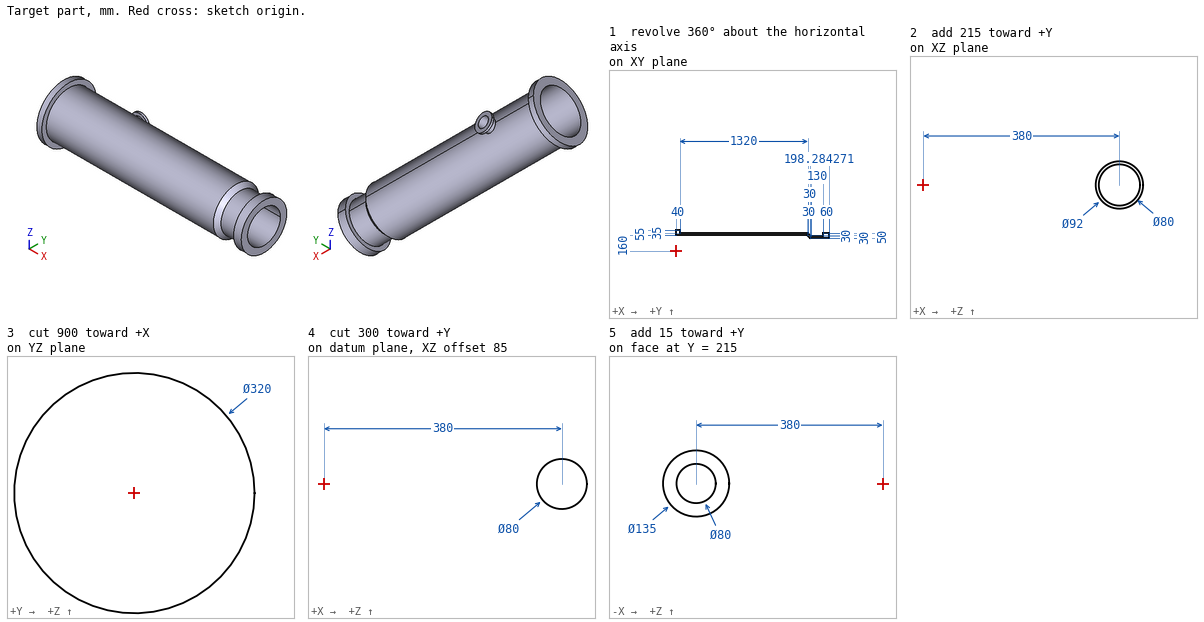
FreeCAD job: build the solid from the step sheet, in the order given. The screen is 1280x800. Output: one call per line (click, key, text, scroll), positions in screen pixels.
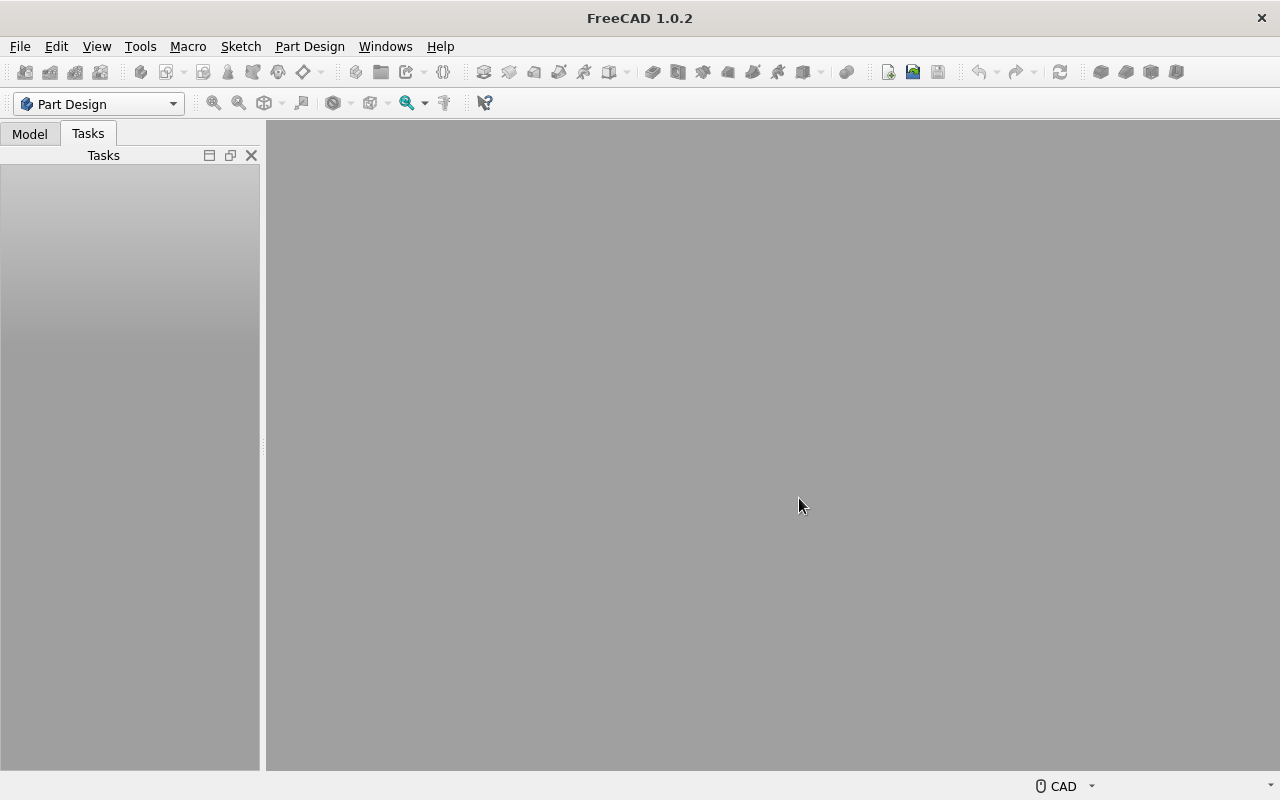
key(ctrl+n)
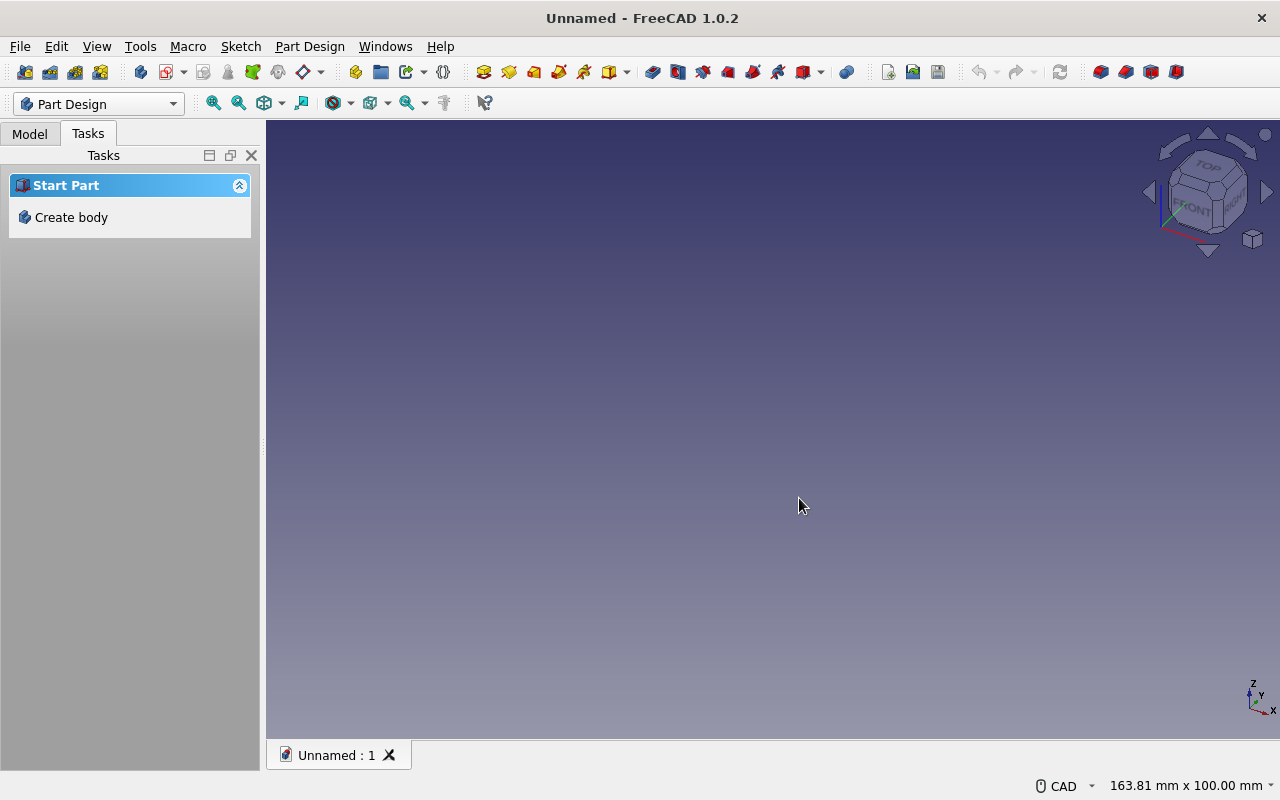
click(166, 72)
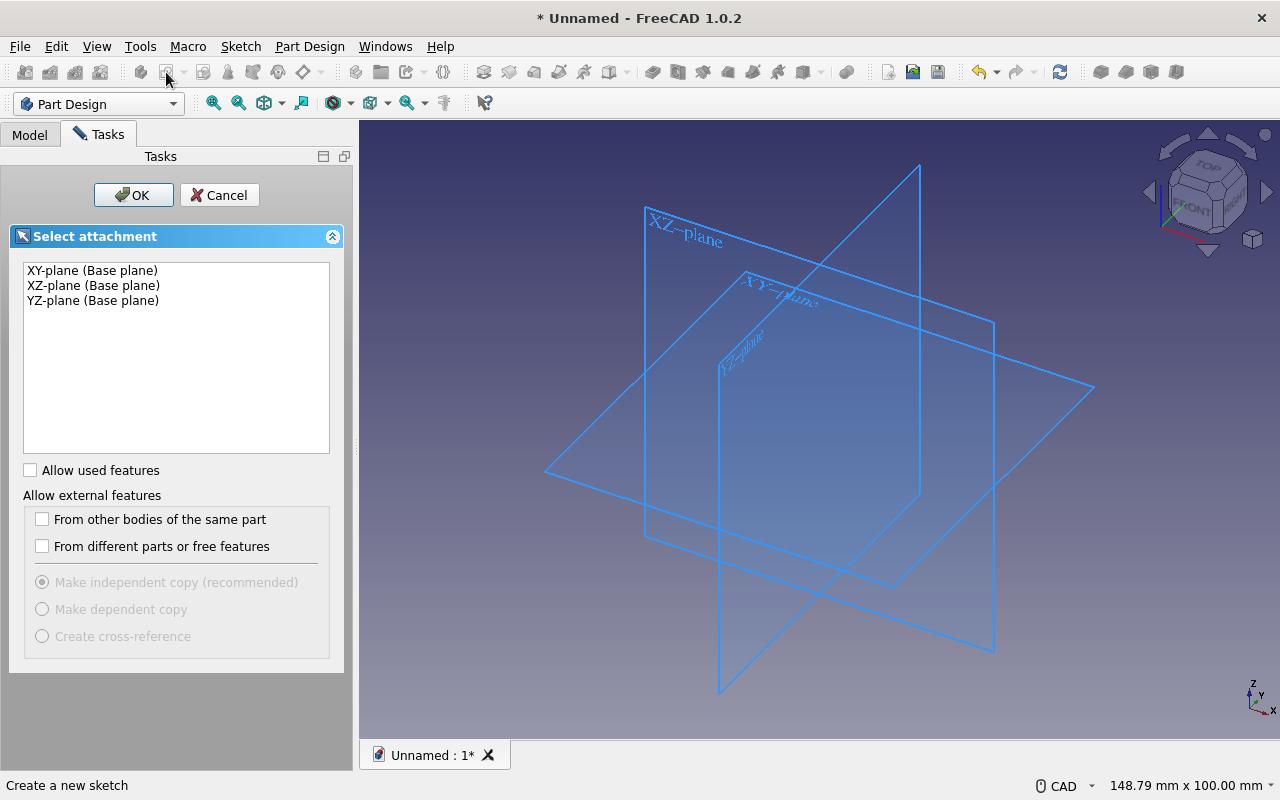
click(84, 270)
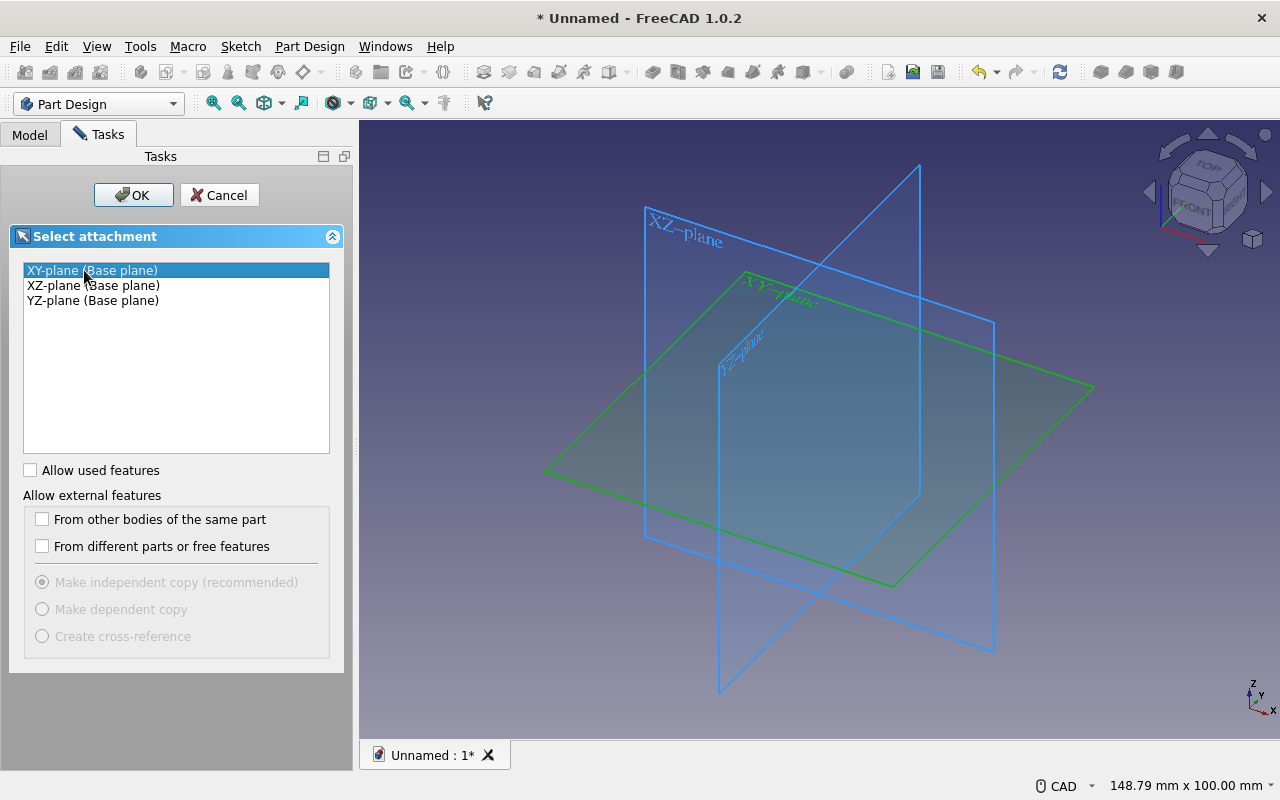
click(134, 195)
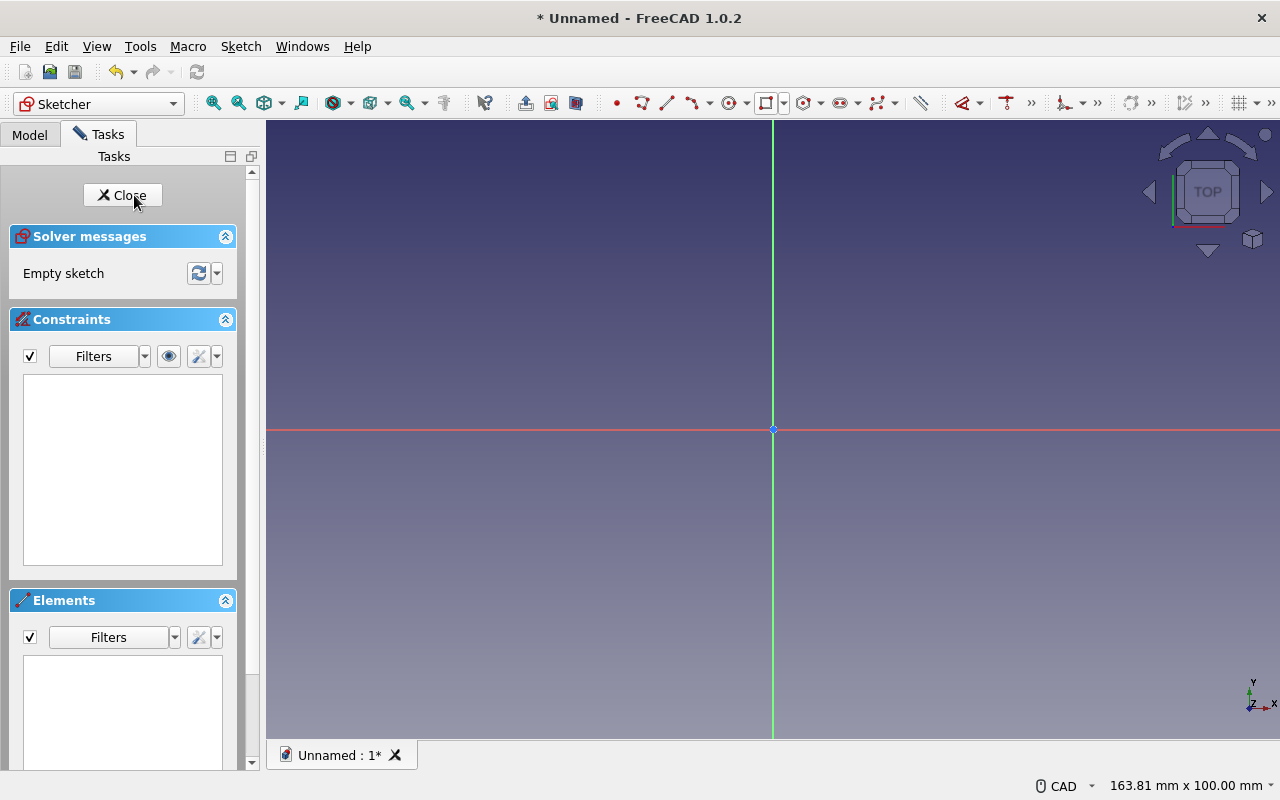
scroll(383, 473, down, 14)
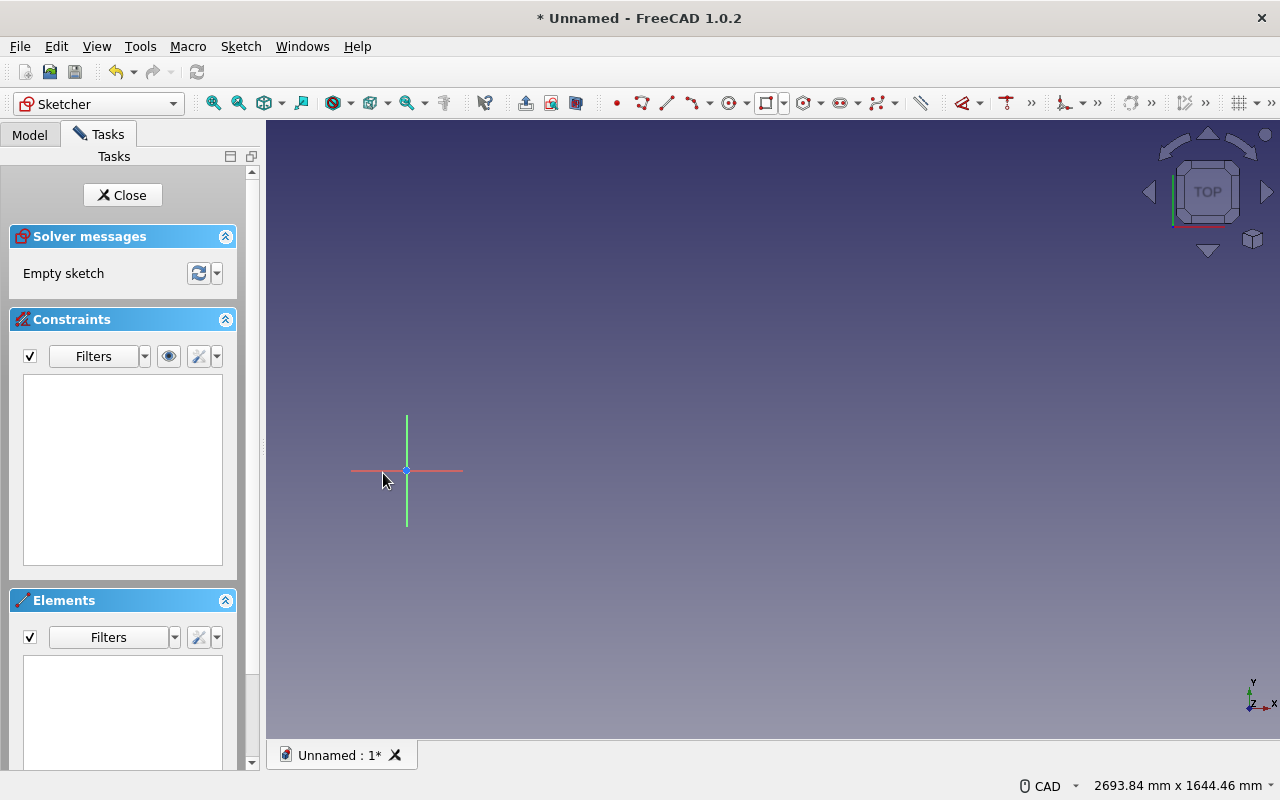
key(g)
key(m)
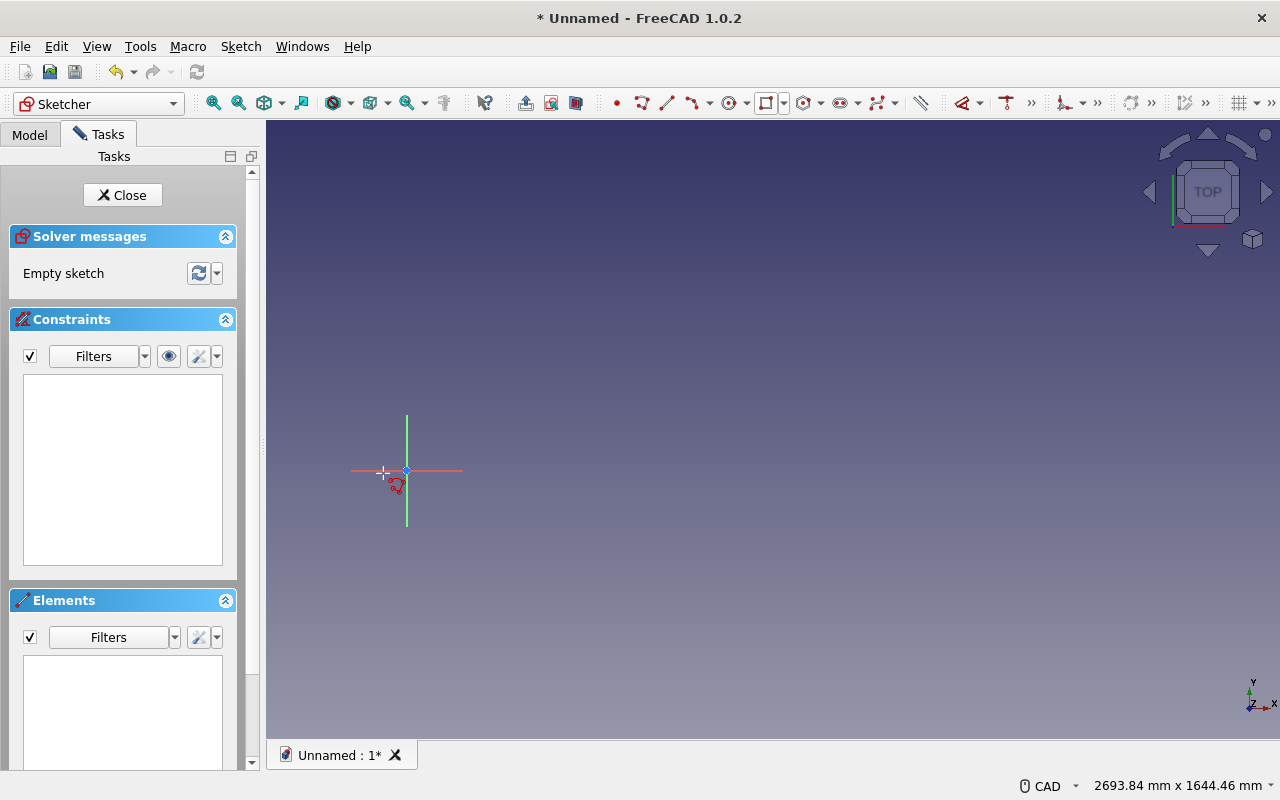
click(407, 411)
click(916, 411)
click(927, 422)
click(1002, 422)
click(1002, 403)
click(979, 403)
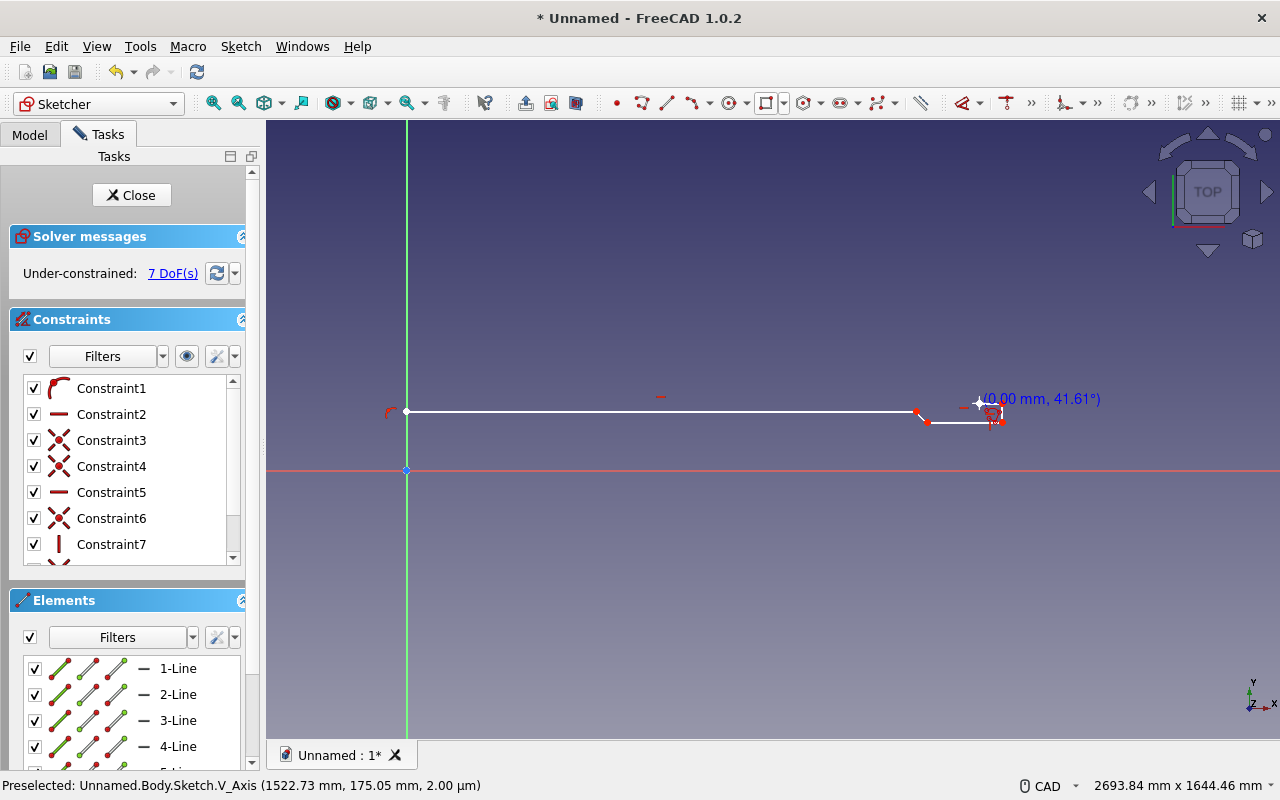
scroll(979, 414, up, 4)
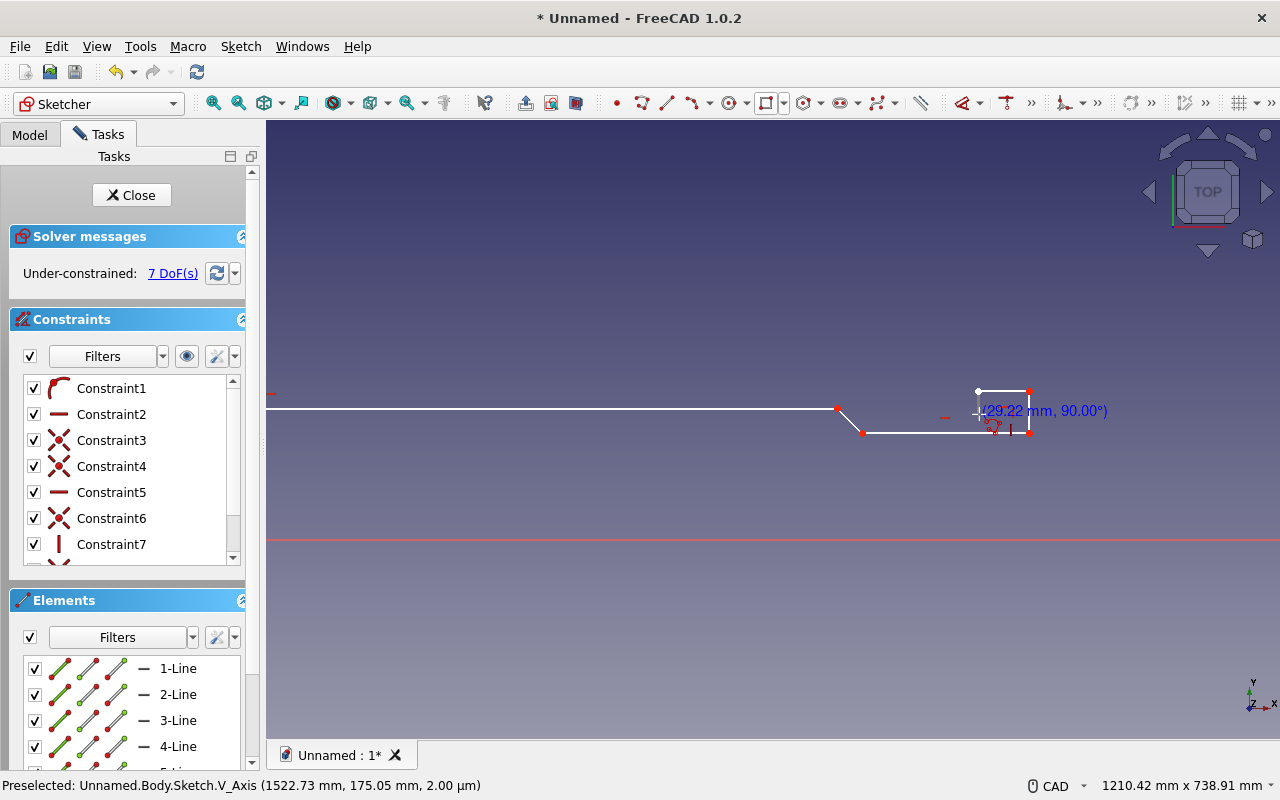
click(978, 414)
click(869, 414)
click(844, 389)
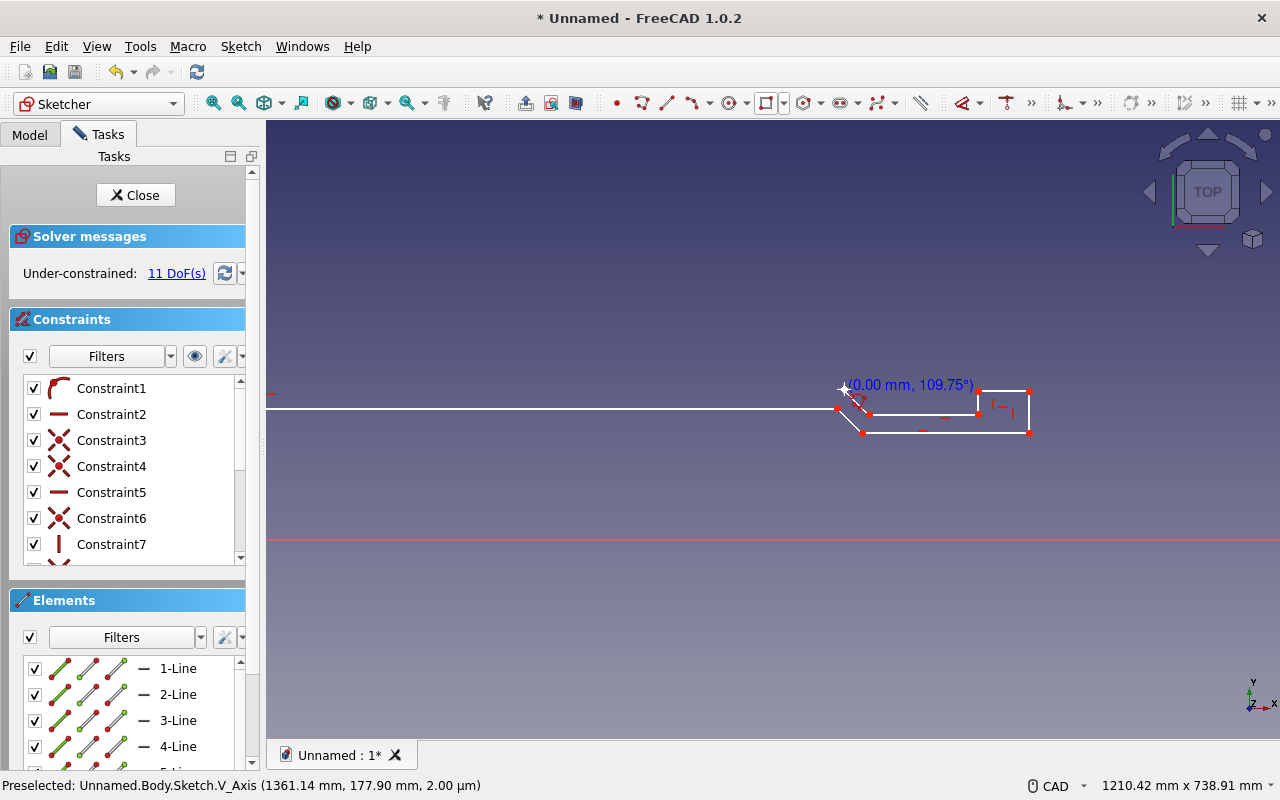
scroll(980, 413, down, 4)